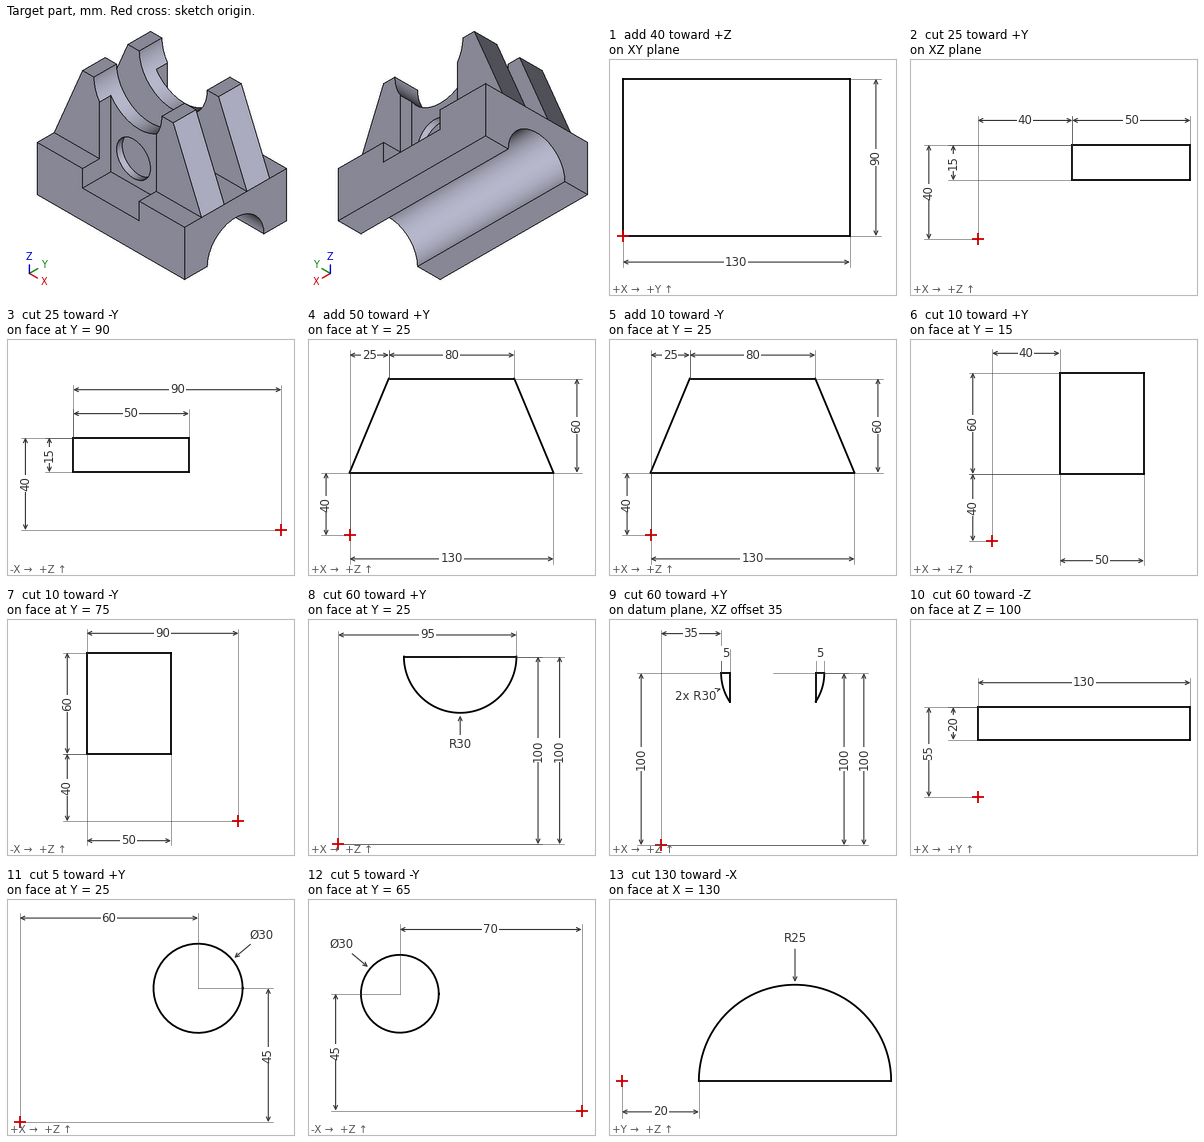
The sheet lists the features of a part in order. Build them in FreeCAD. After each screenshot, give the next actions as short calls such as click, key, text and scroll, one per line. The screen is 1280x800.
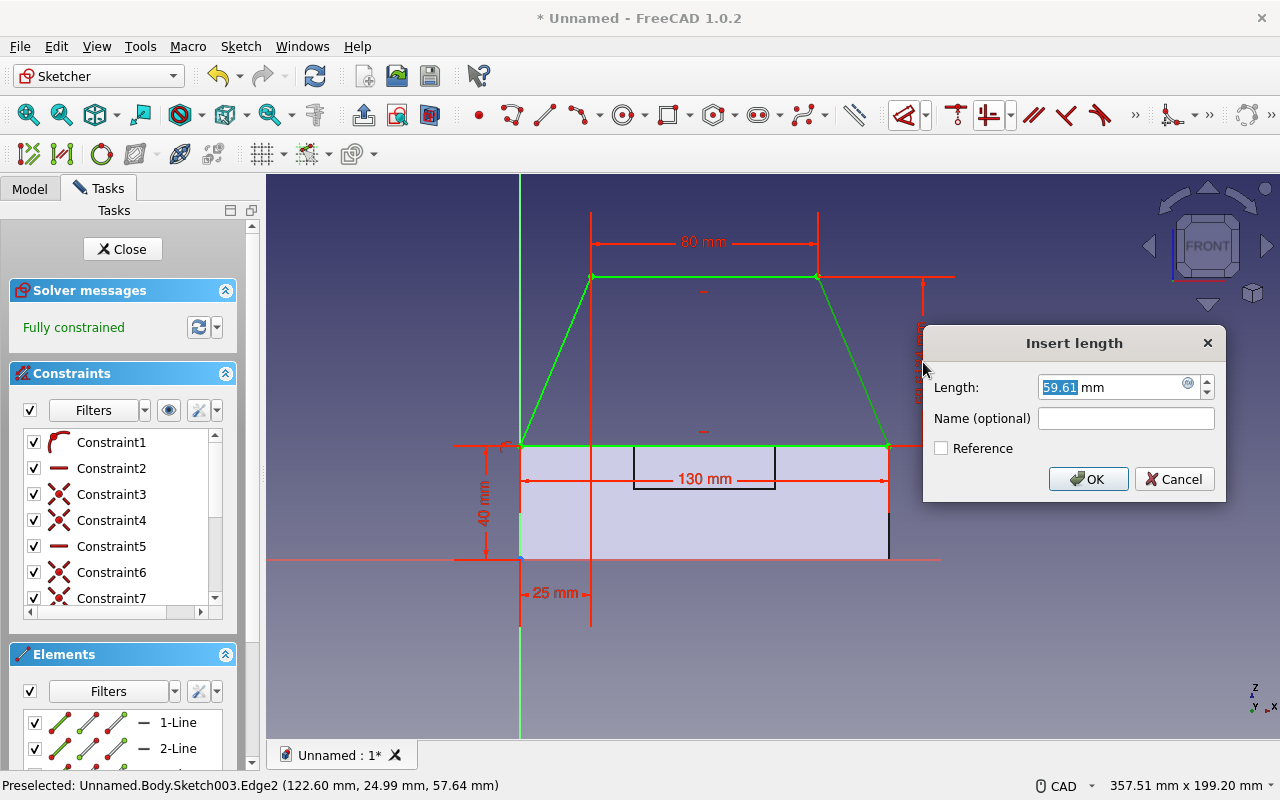
text(60)
key(Return)
key(Escape)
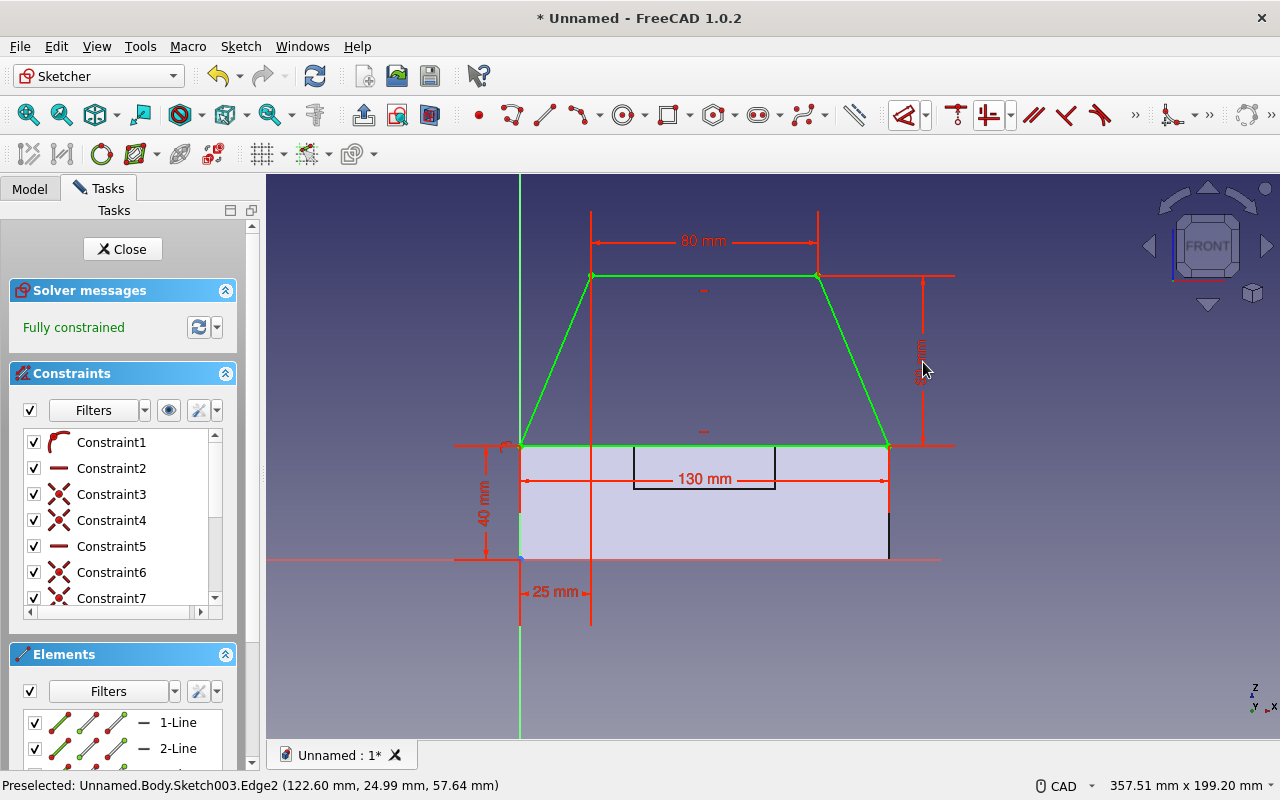
click(123, 249)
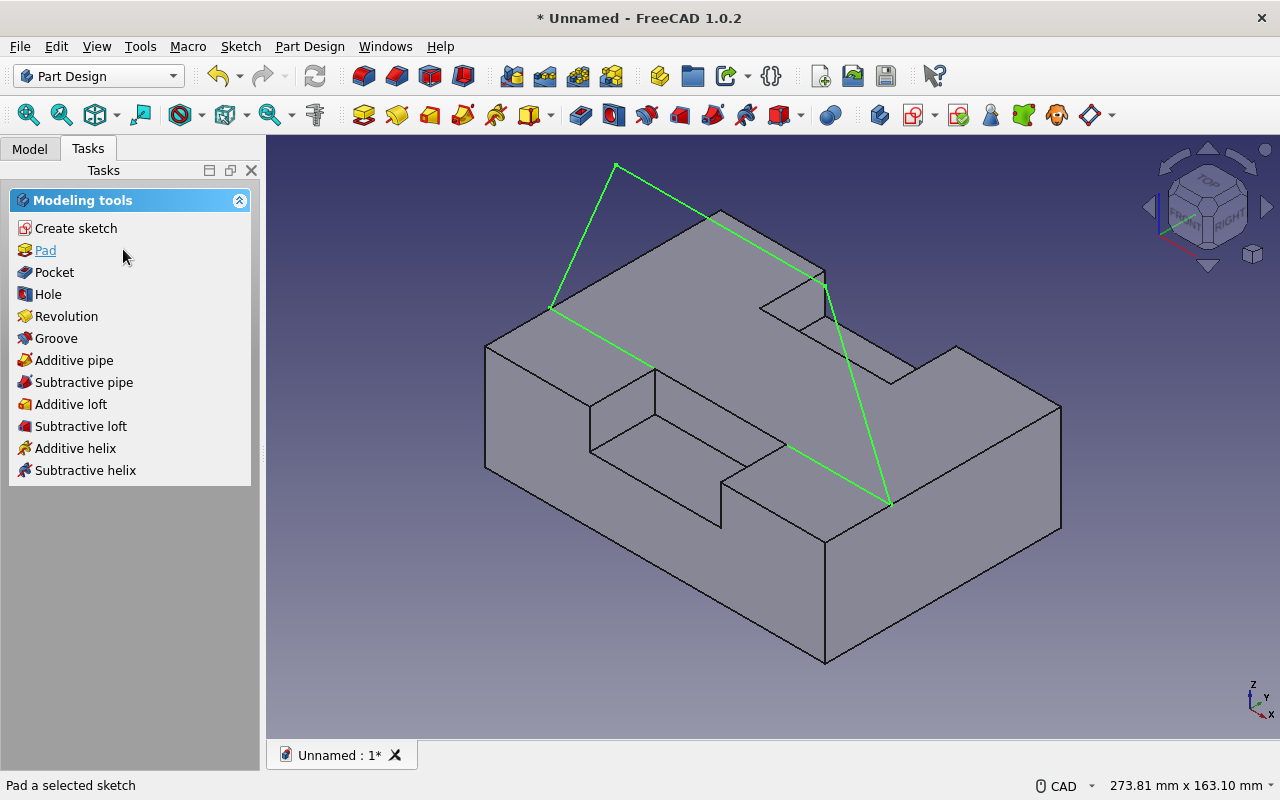
click(364, 116)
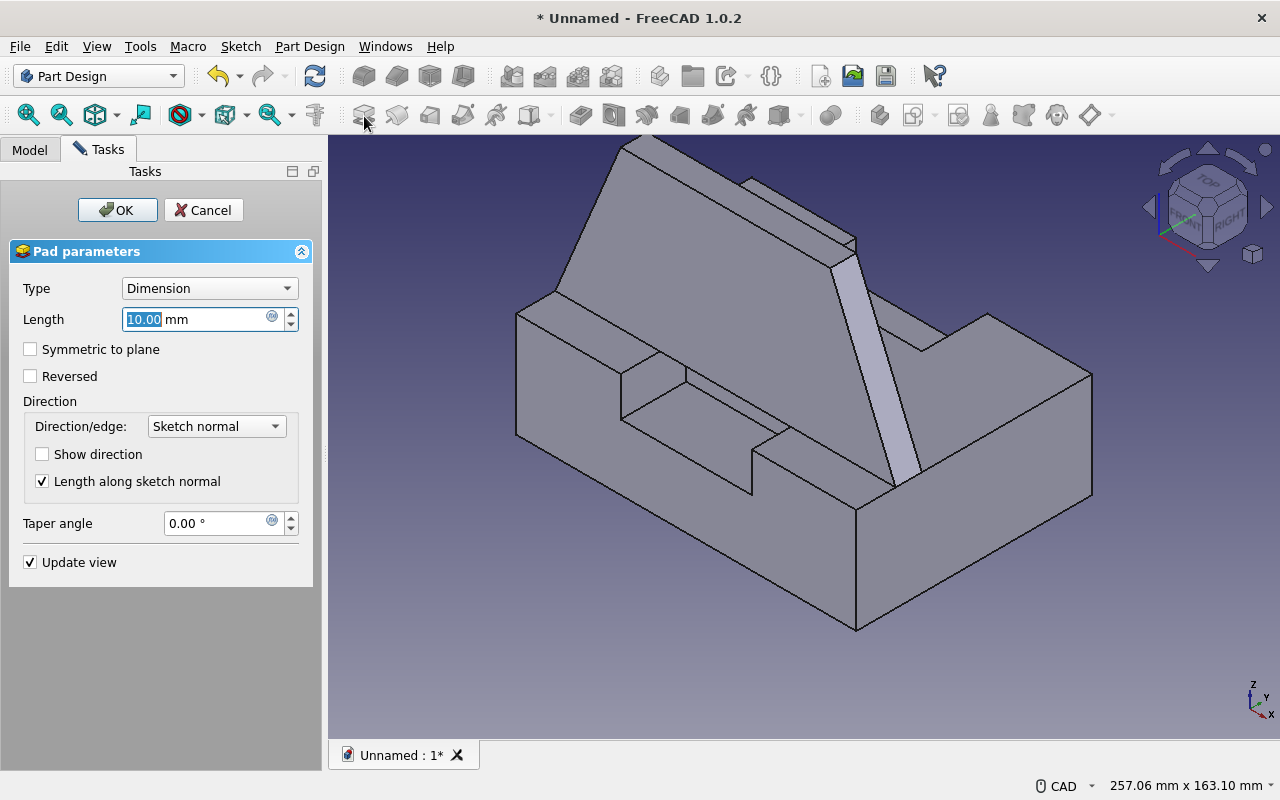
text(50)
key(Tab)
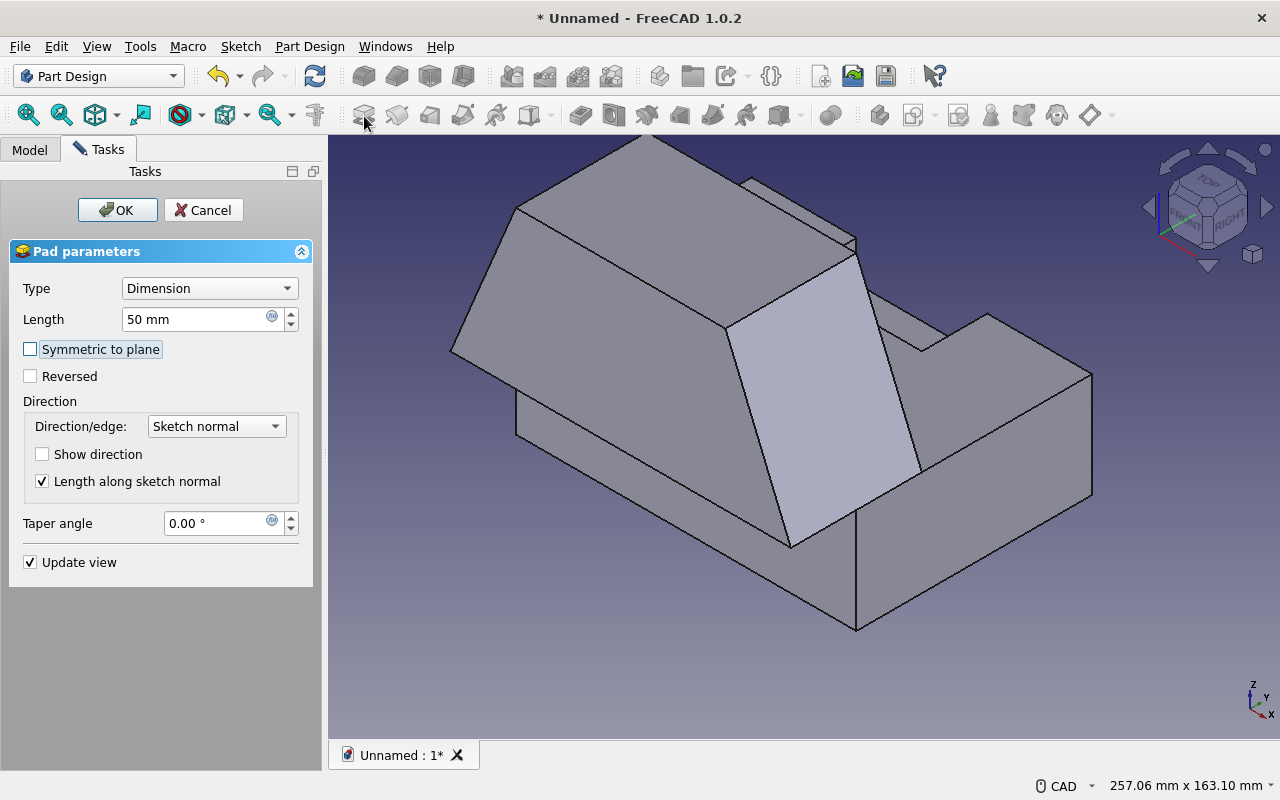
click(31, 376)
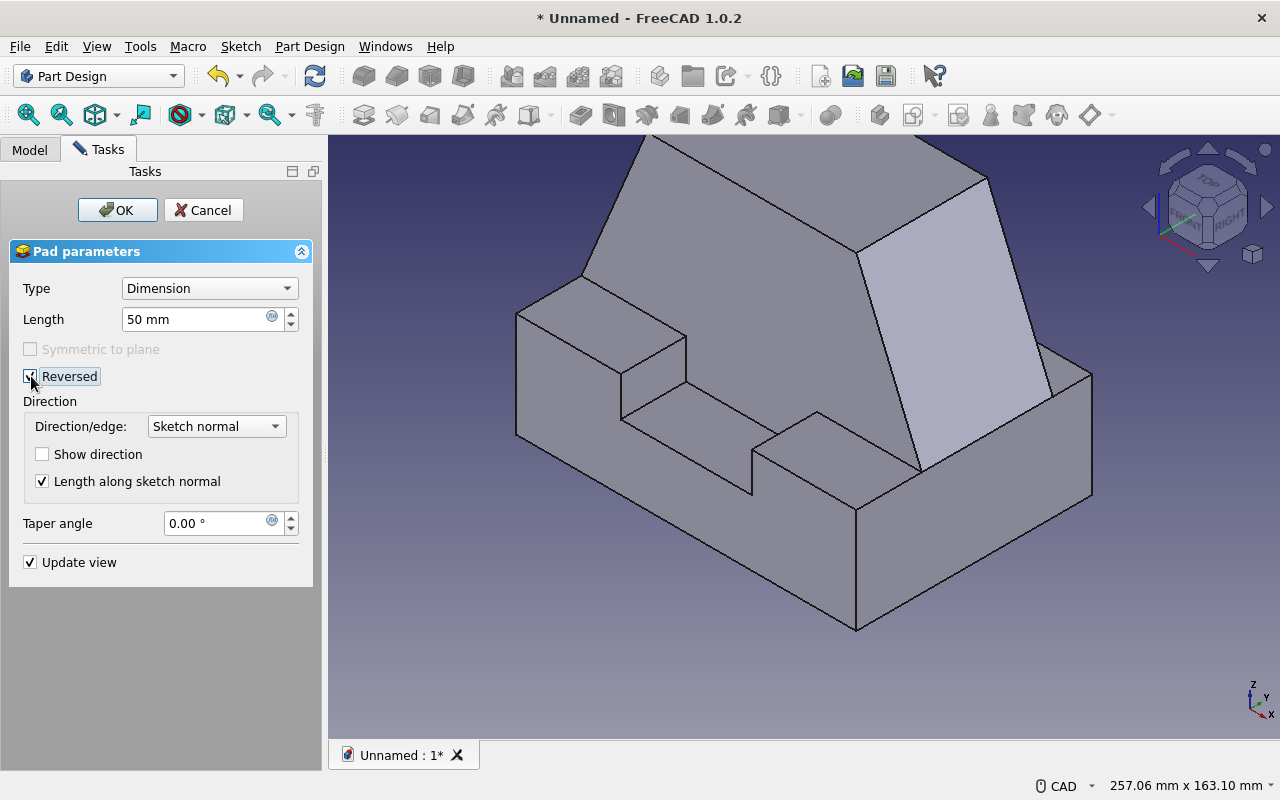
click(118, 210)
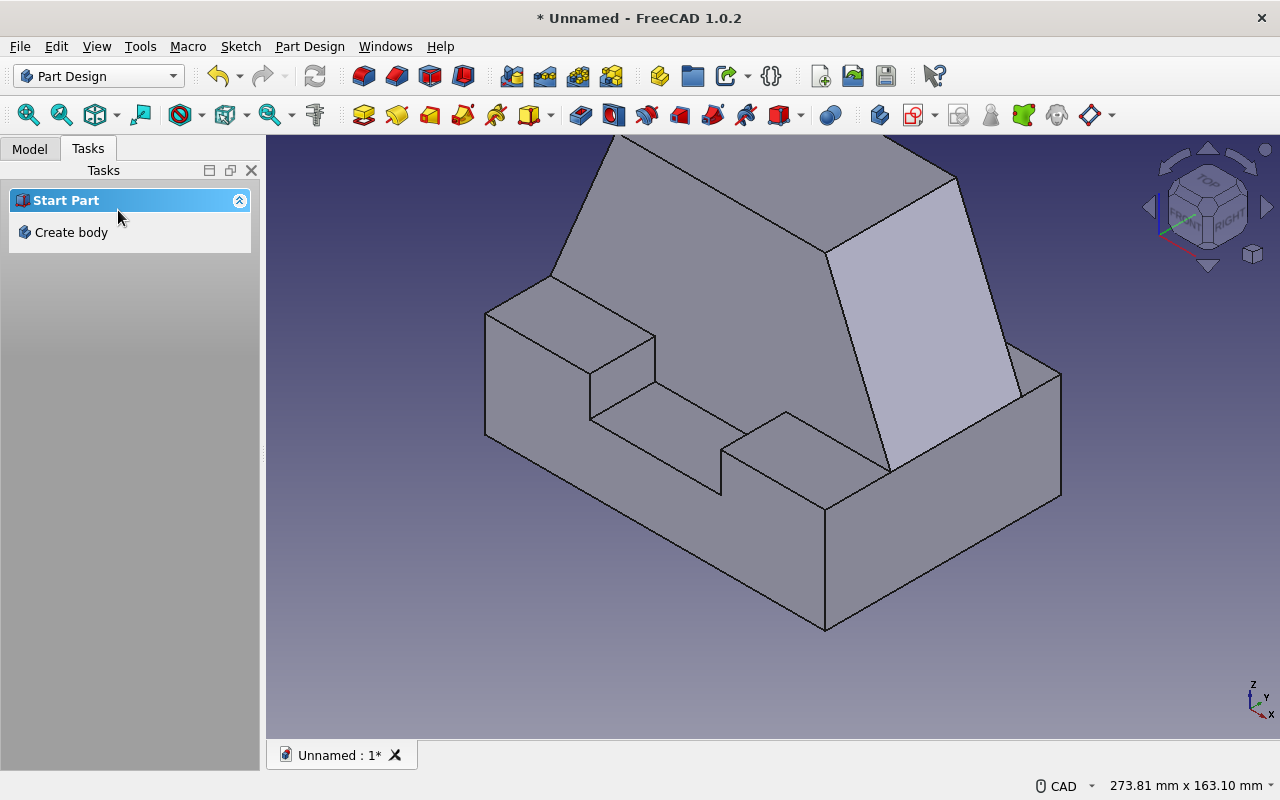
key(v)
key(f)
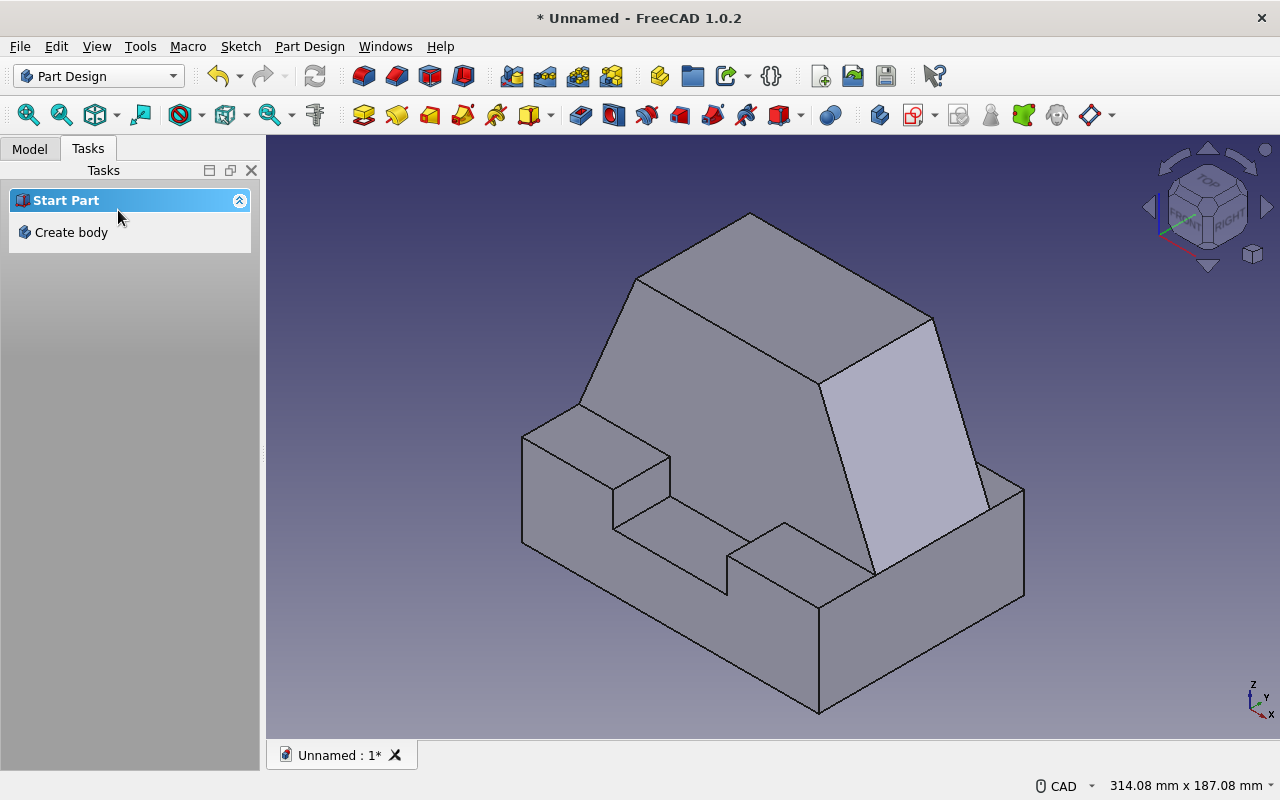
click(727, 429)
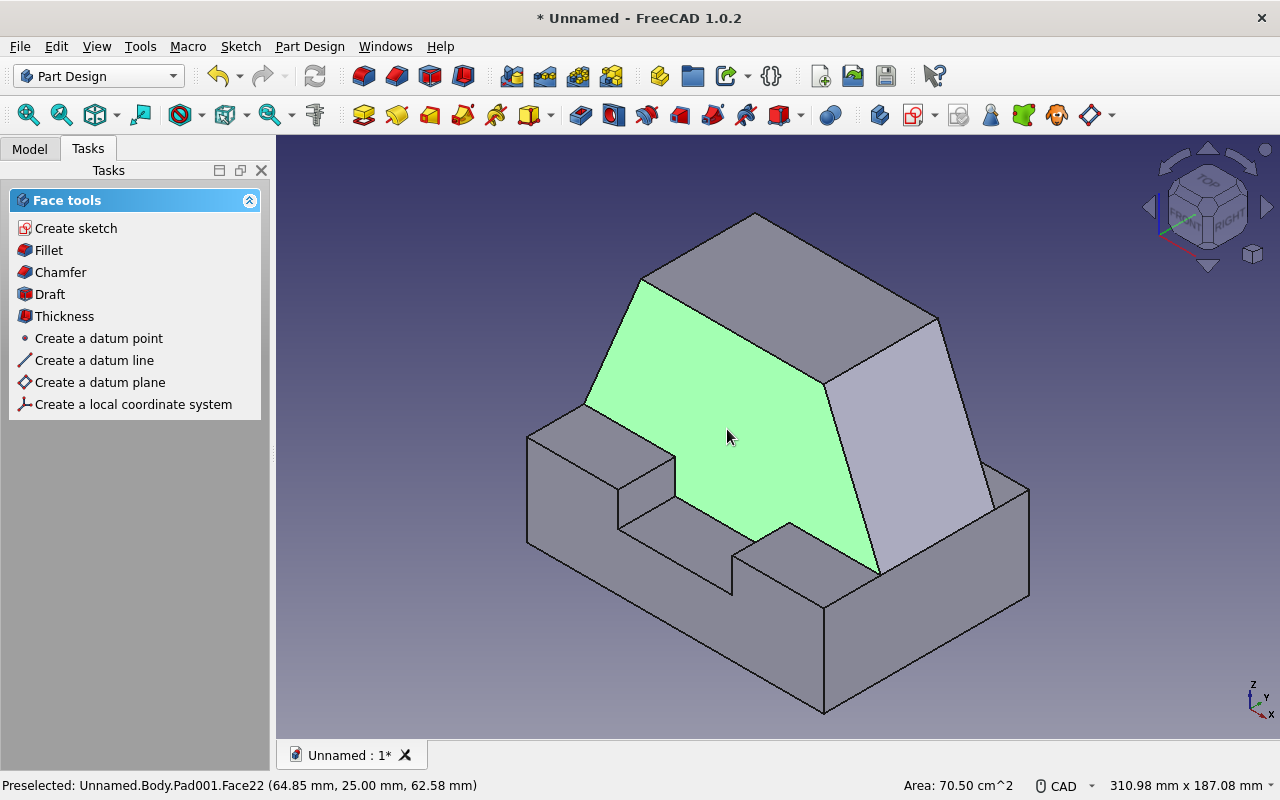
click(912, 116)